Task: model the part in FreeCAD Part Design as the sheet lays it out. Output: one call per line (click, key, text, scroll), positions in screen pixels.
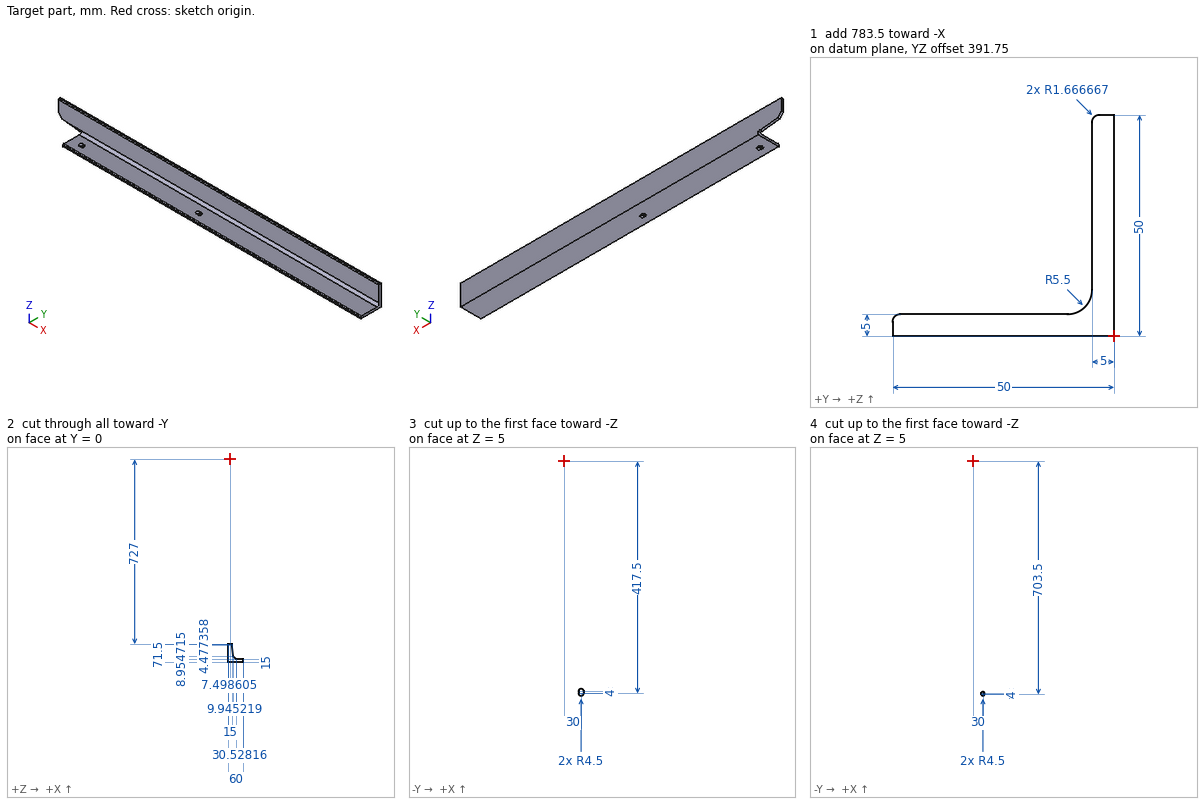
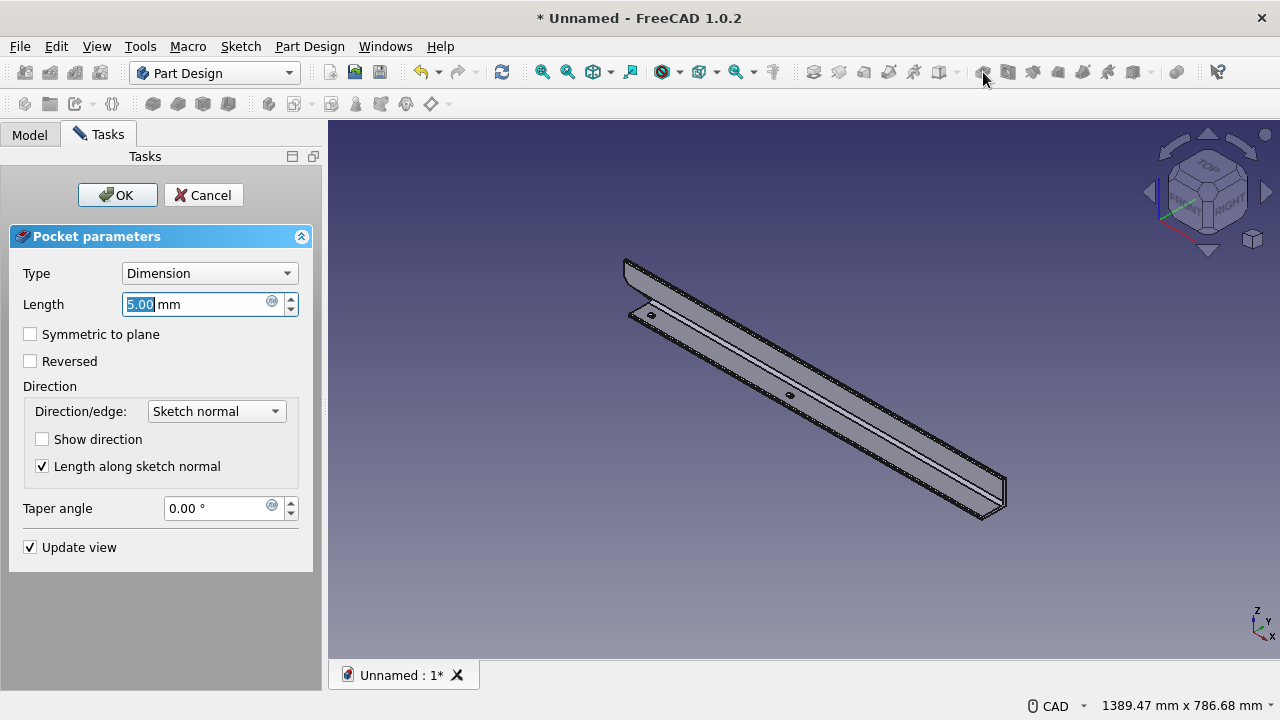
click(210, 274)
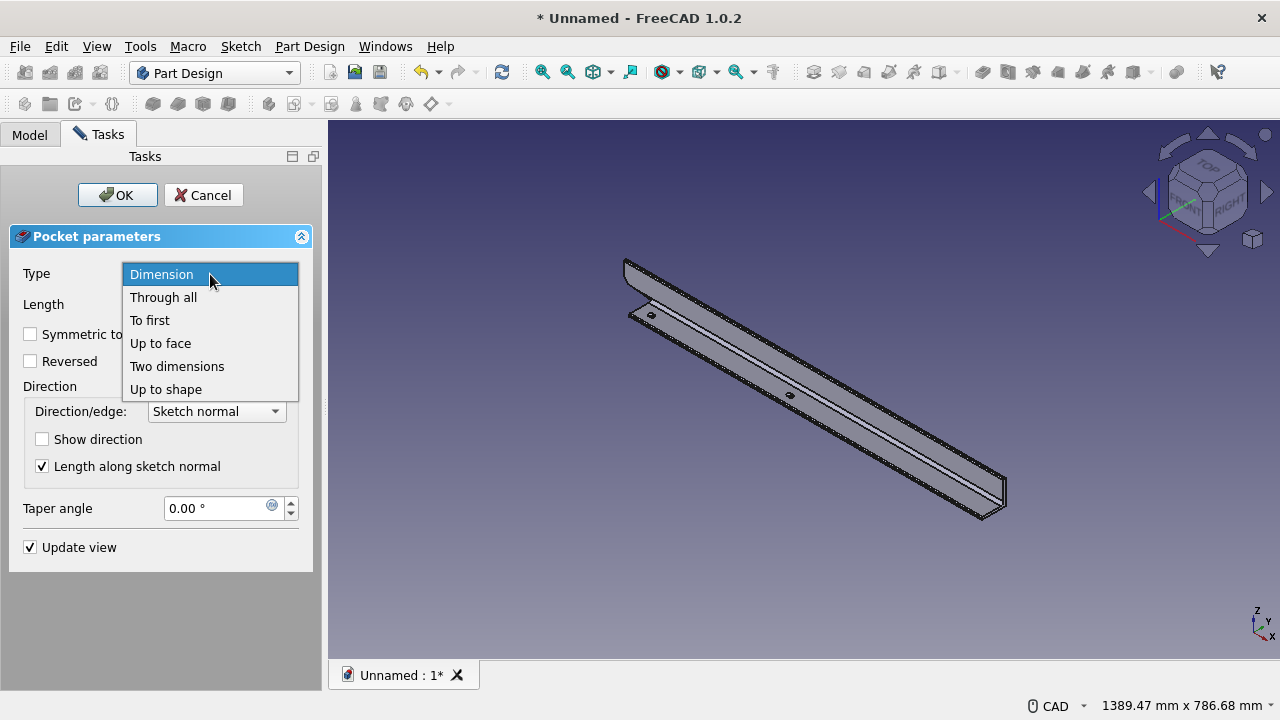
click(208, 320)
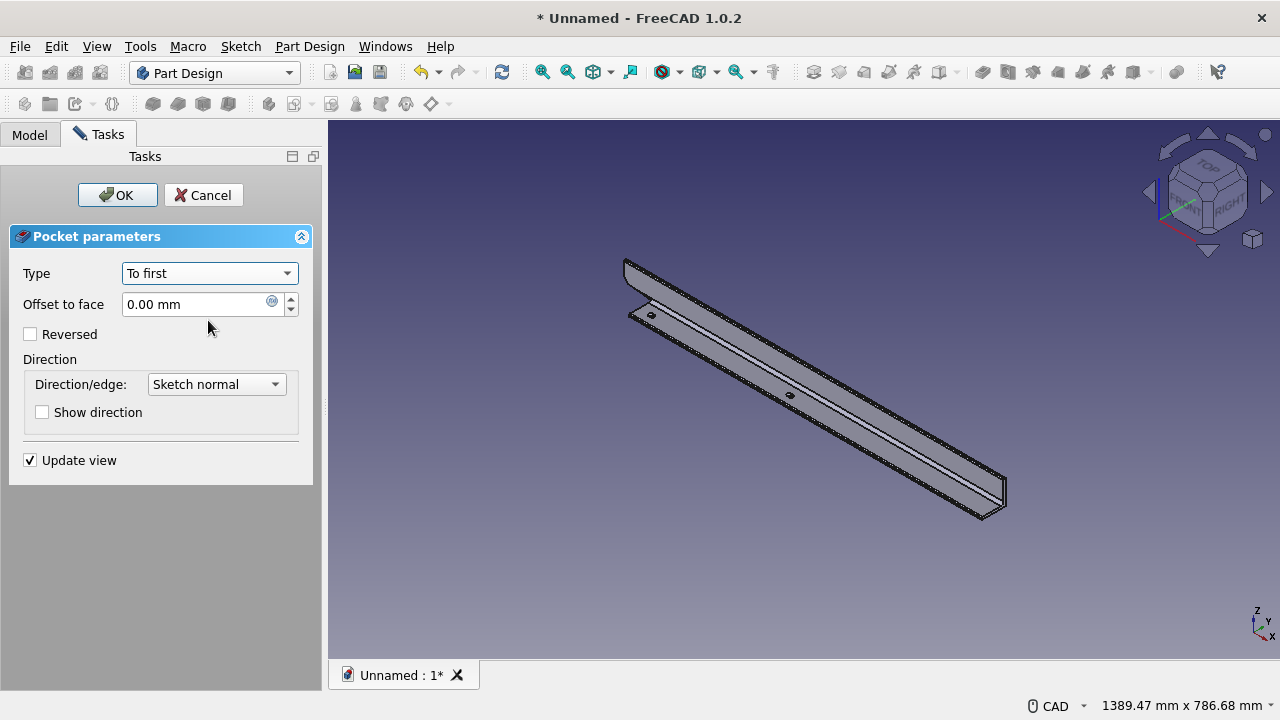
click(118, 195)